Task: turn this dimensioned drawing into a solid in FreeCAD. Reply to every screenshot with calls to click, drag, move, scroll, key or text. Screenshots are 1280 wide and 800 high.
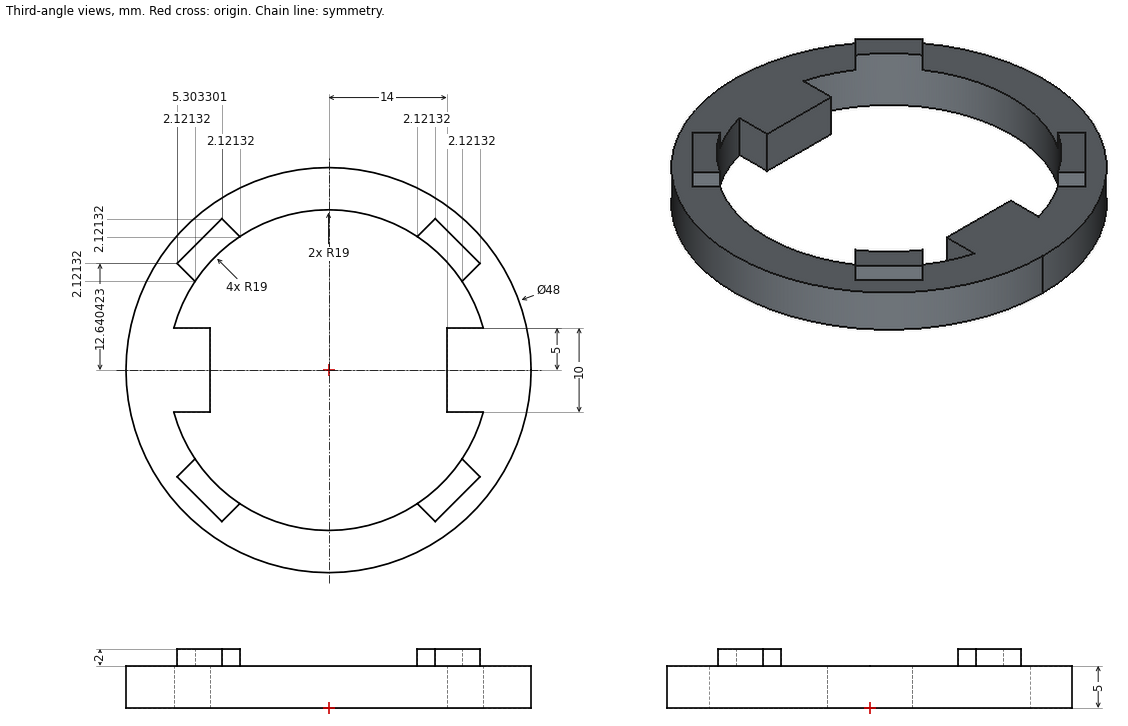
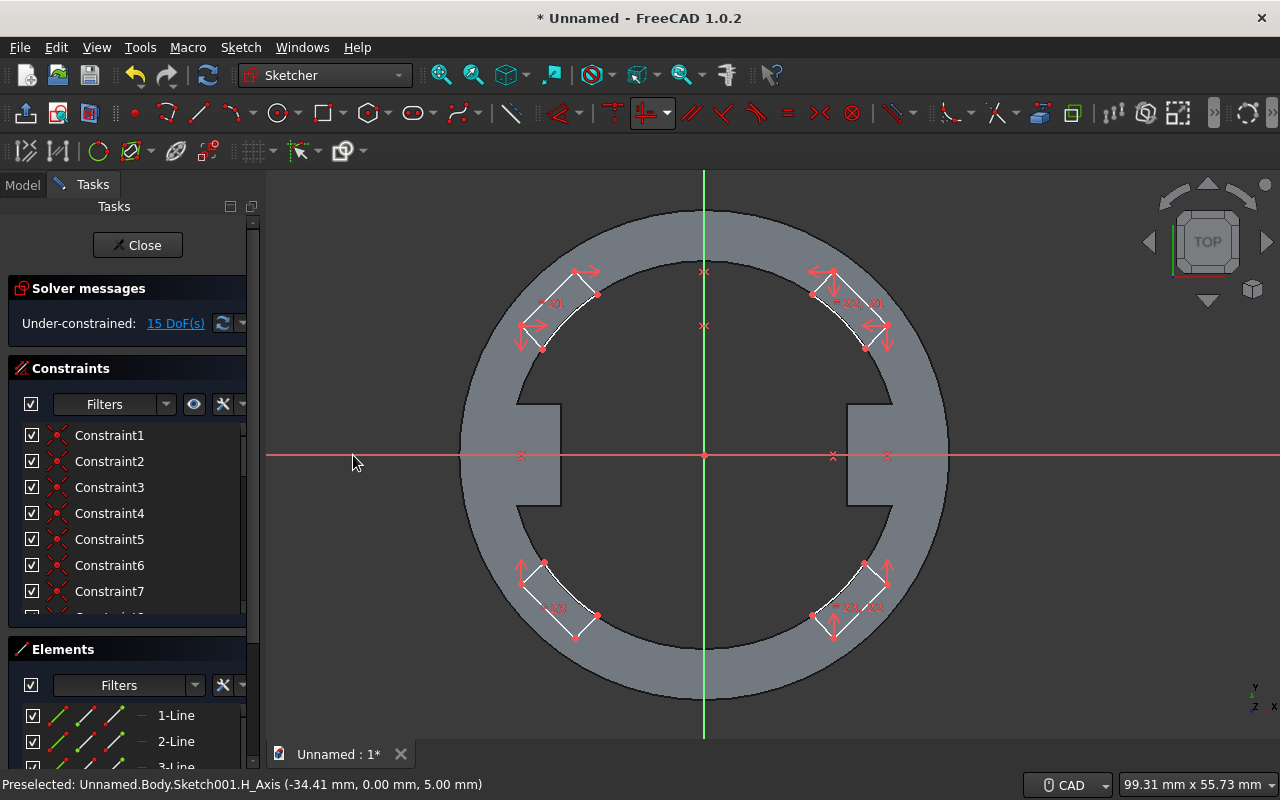
click(575, 272)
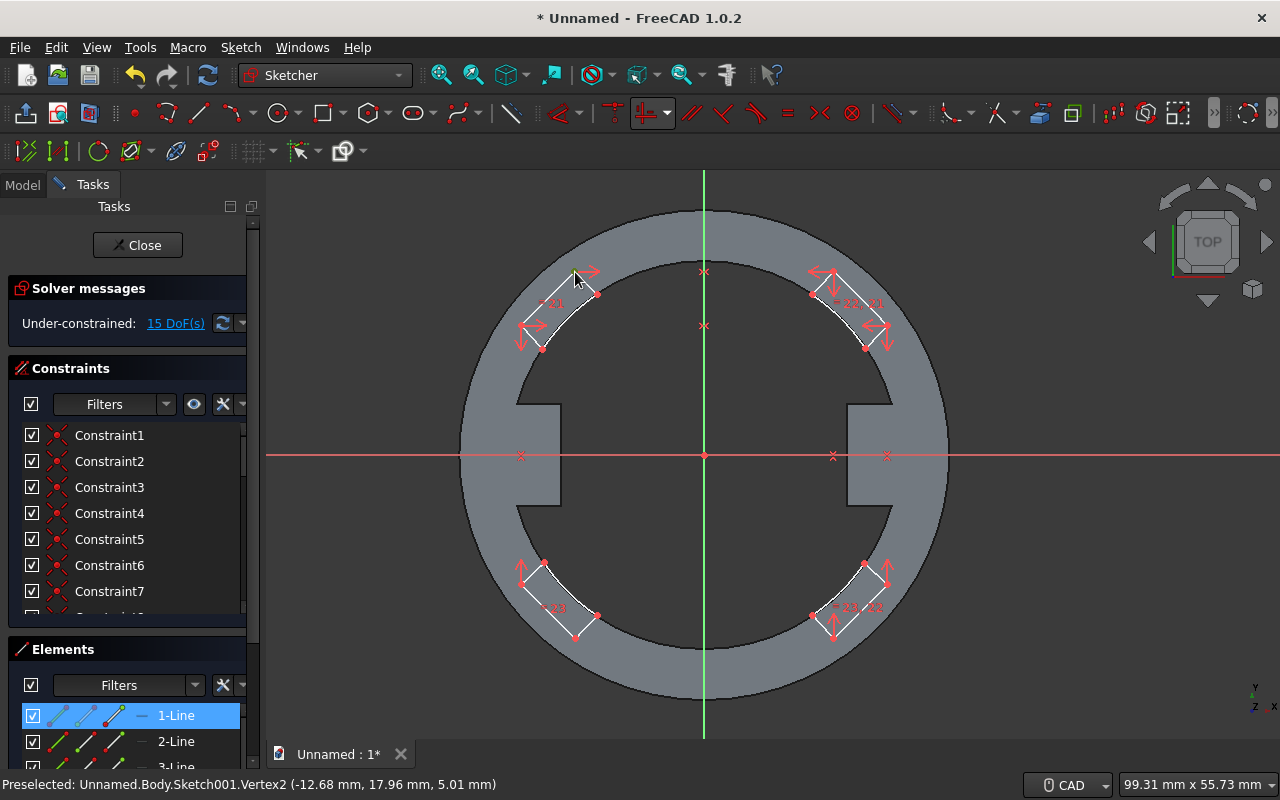
click(575, 639)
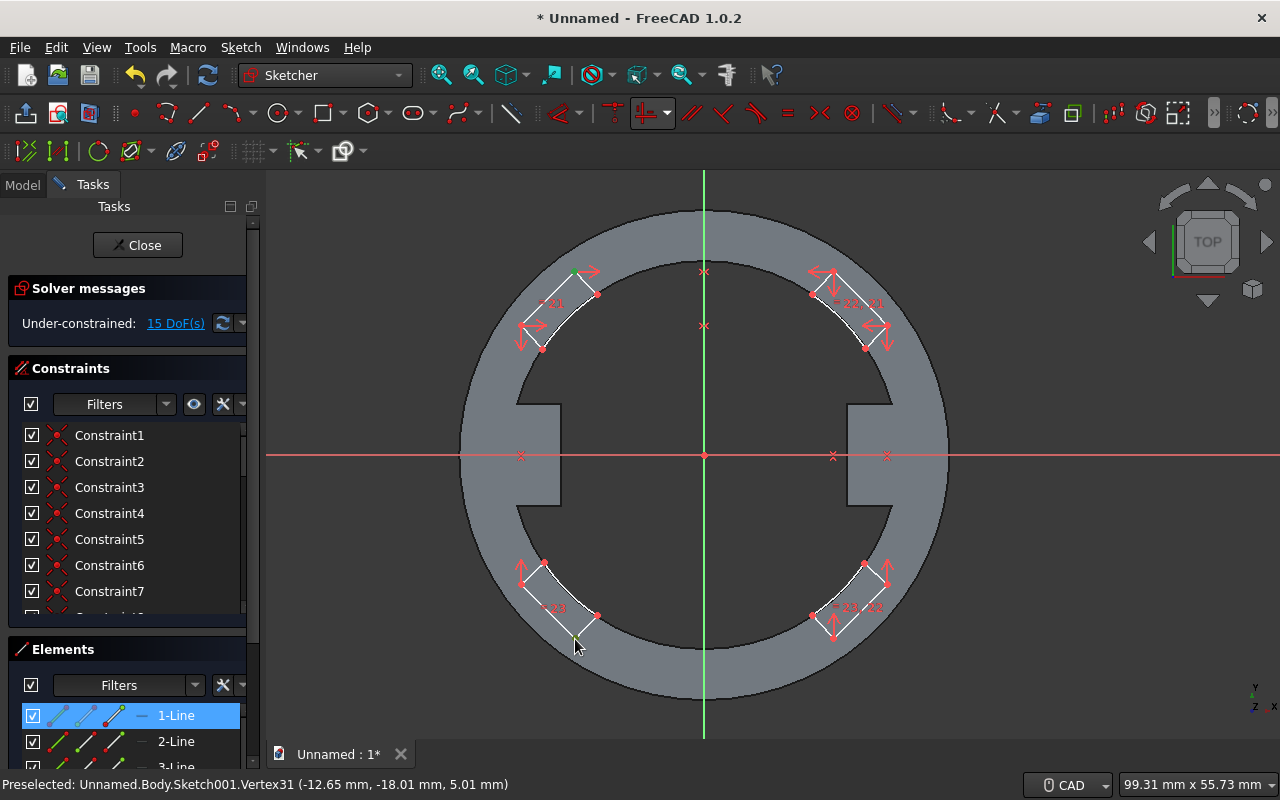
click(353, 455)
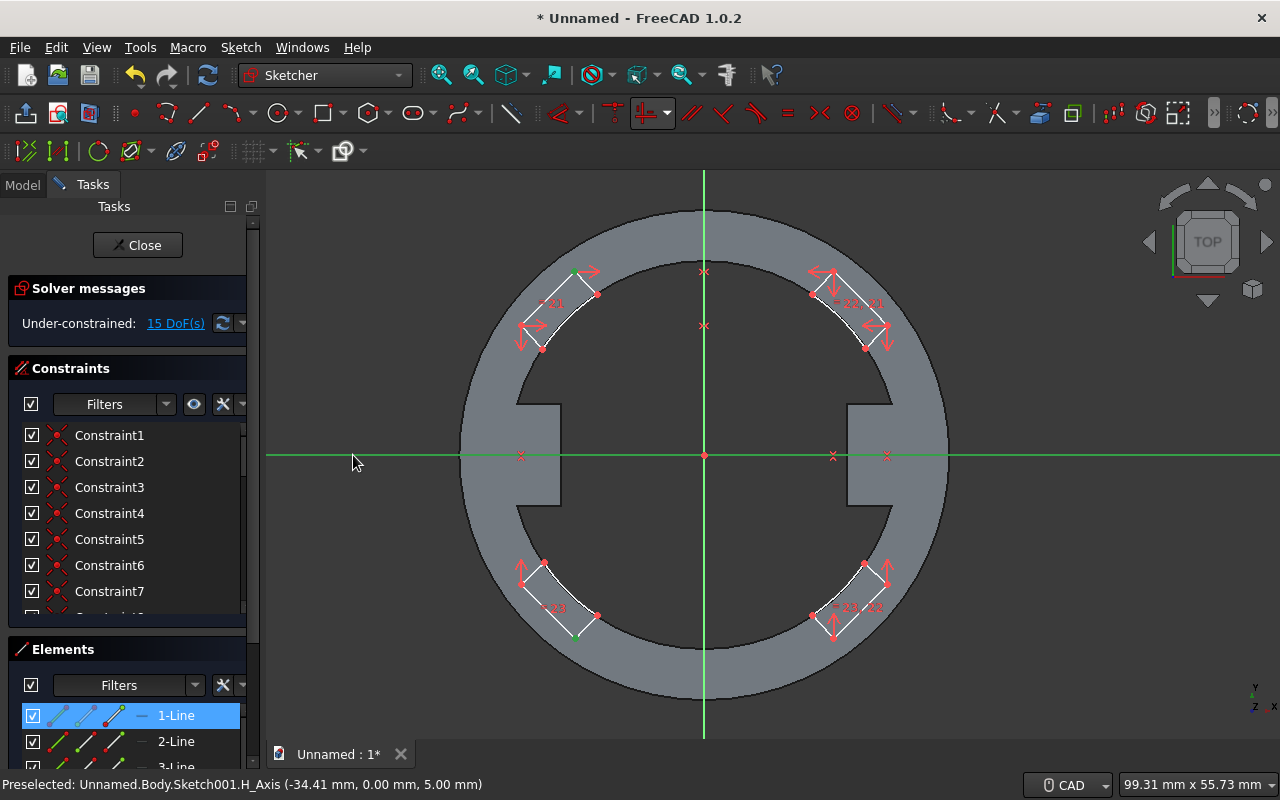
key(s)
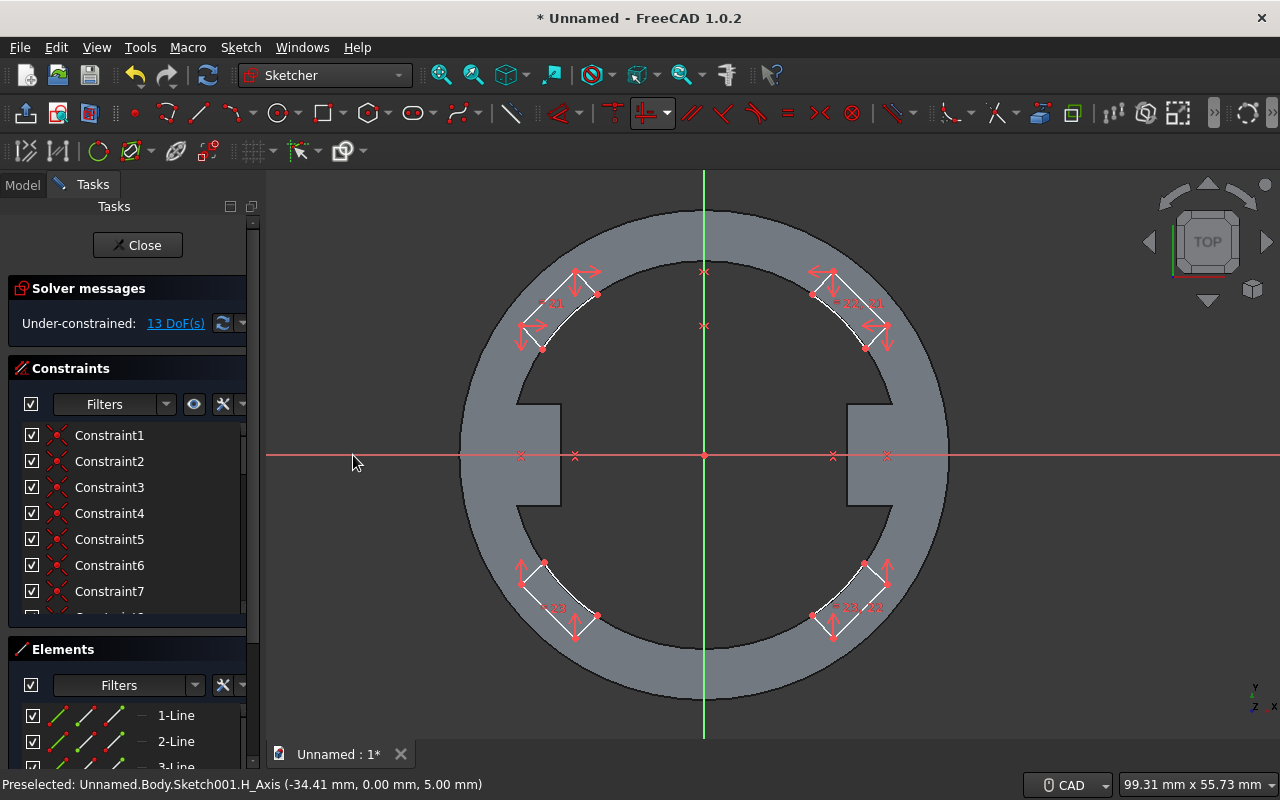
key(d)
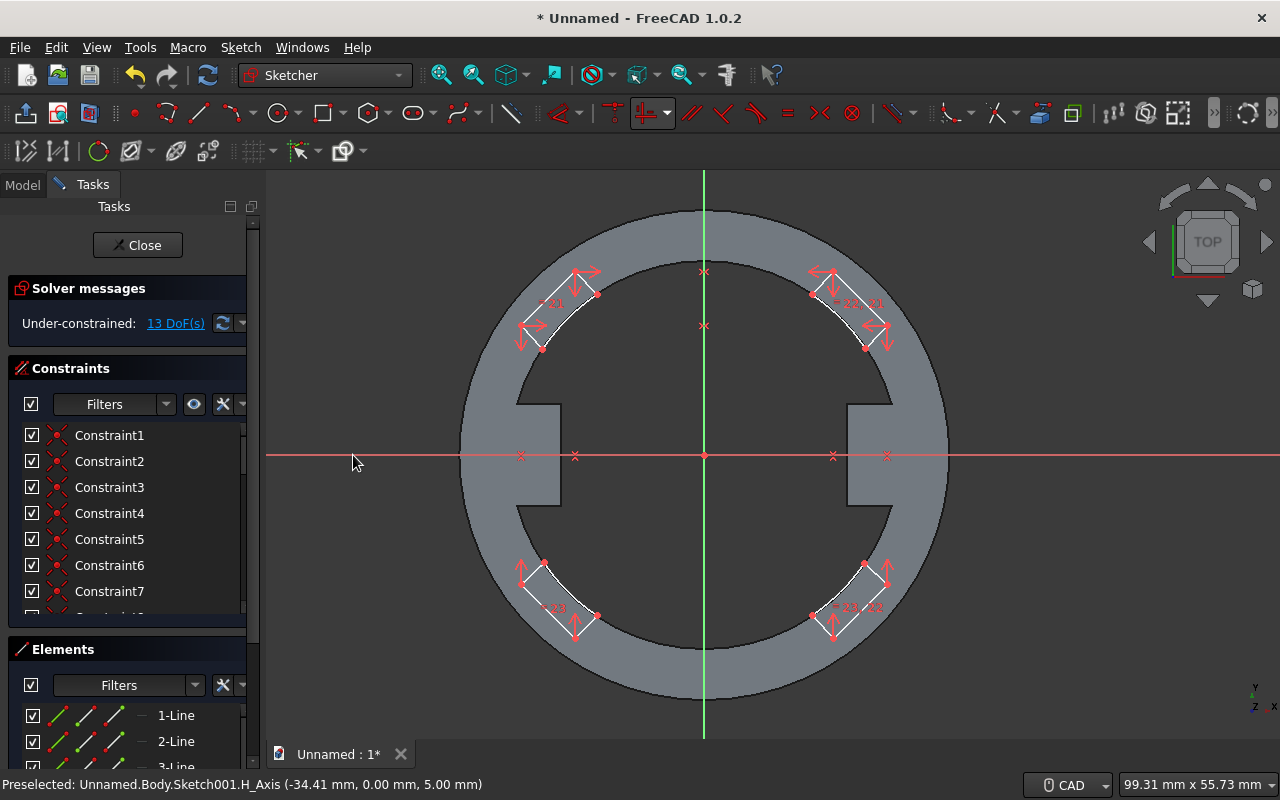
click(578, 309)
click(657, 235)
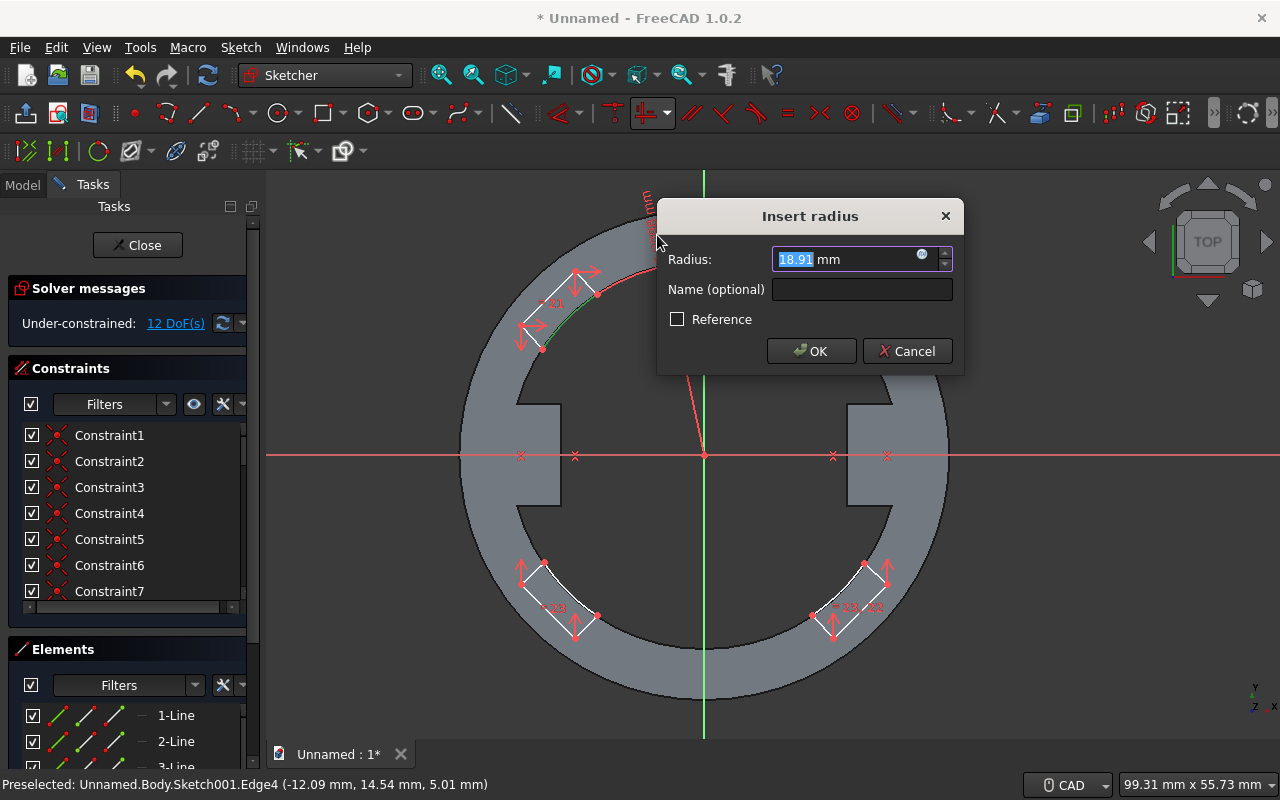
text(19)
key(Return)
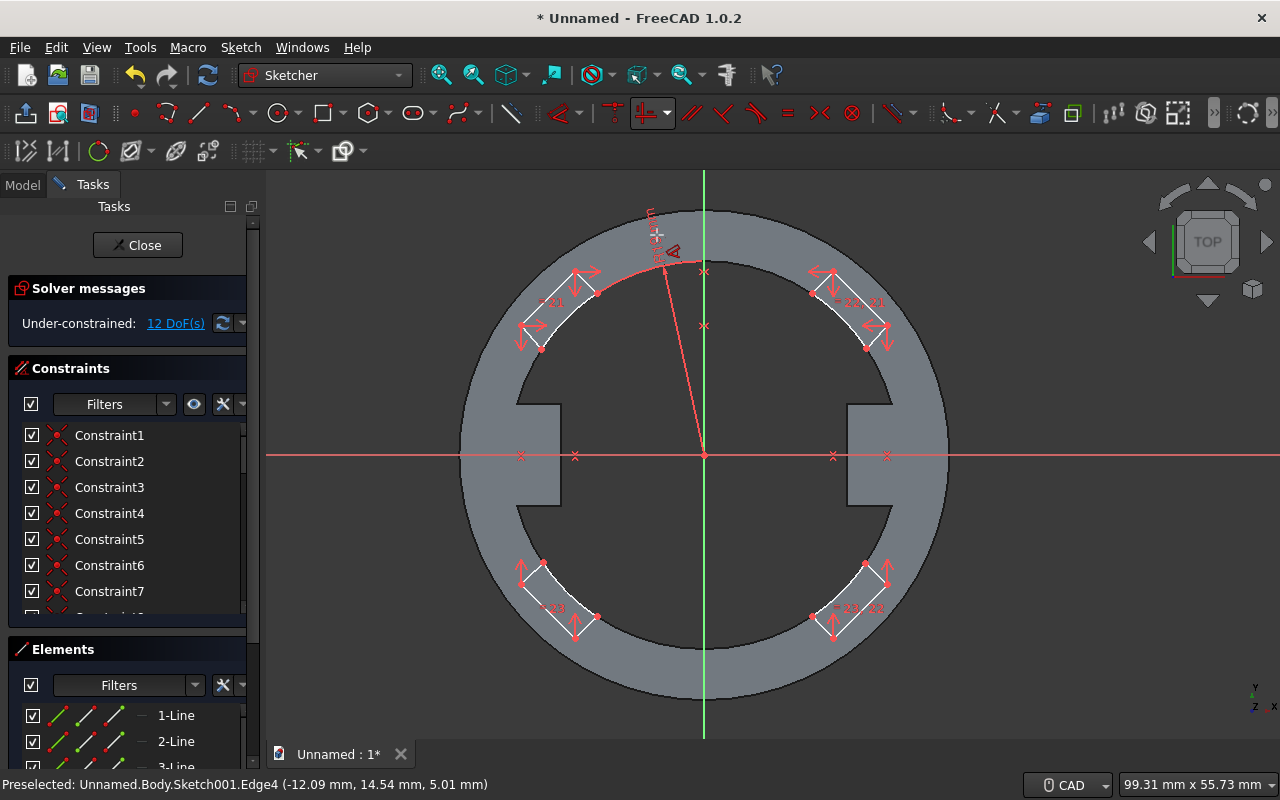
scroll(591, 287, up, 4)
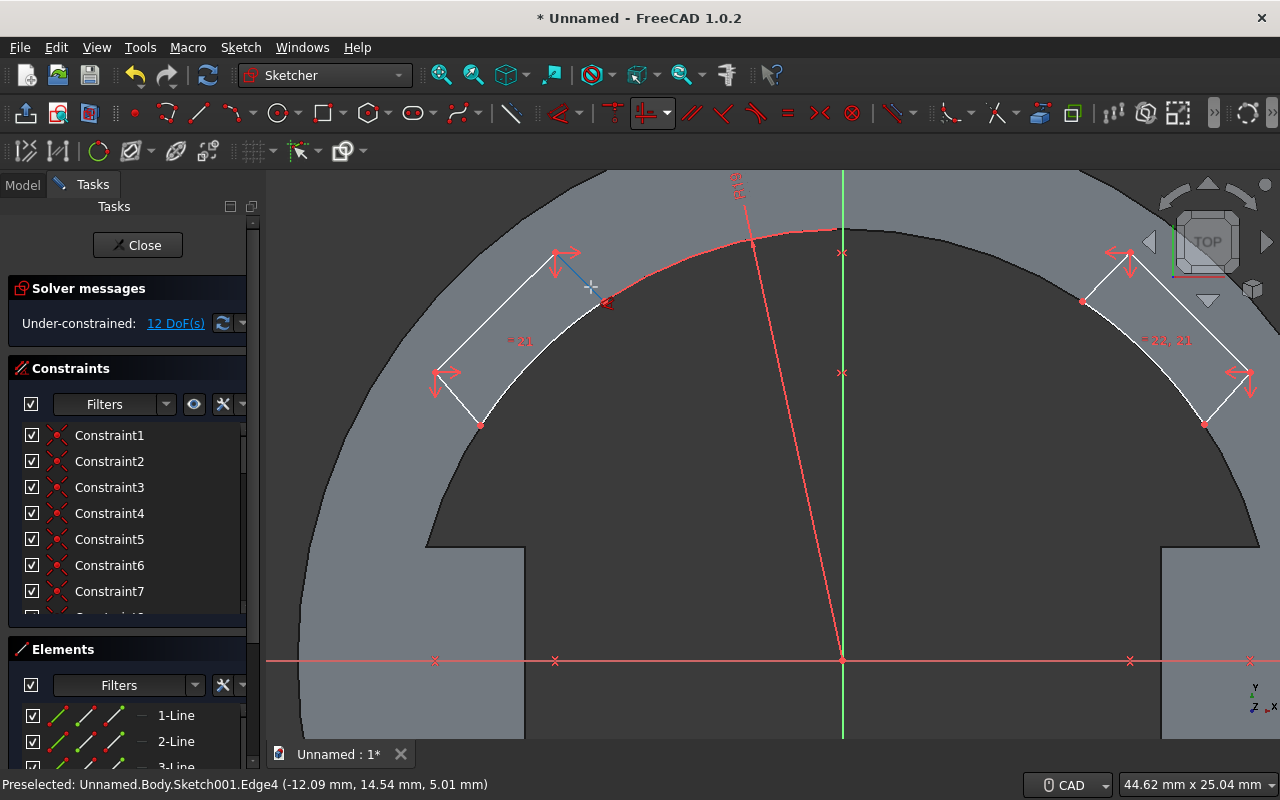
click(589, 287)
click(580, 219)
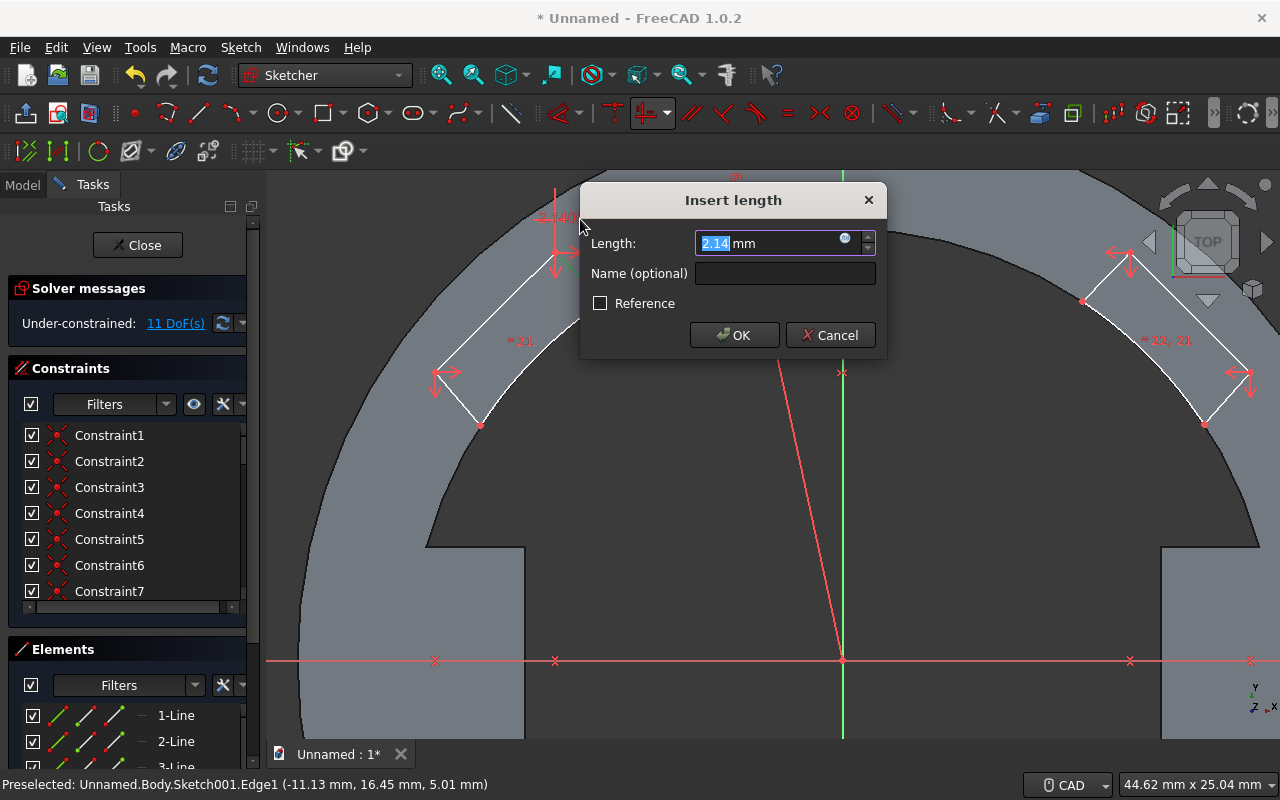
text(2.12132)
key(Return)